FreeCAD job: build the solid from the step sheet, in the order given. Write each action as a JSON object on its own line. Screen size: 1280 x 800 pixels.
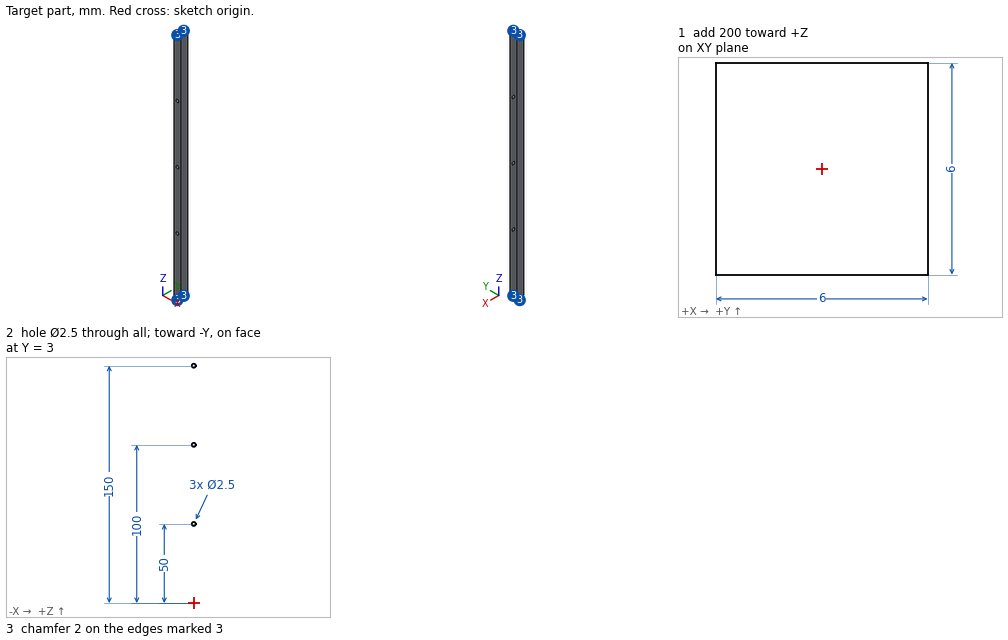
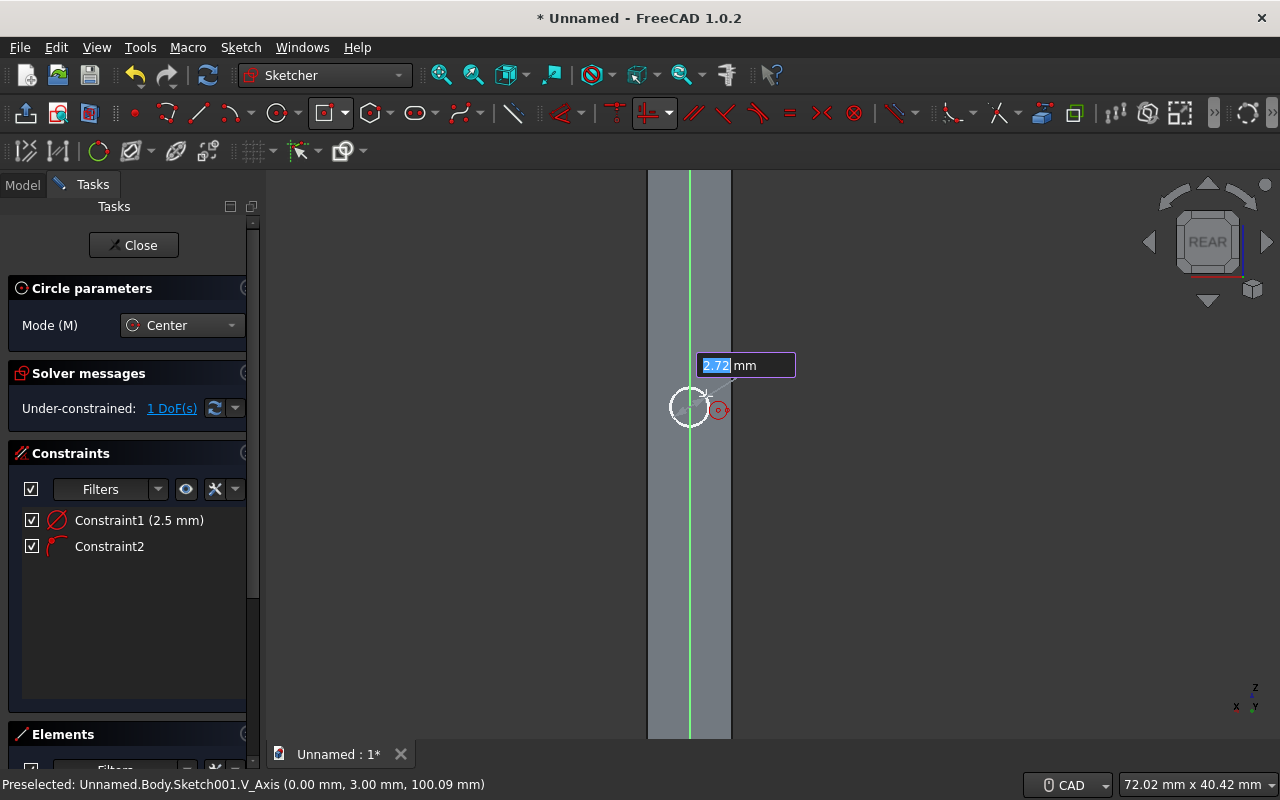
{"action": "type", "text": "2.5"}
{"action": "key", "text": "Return"}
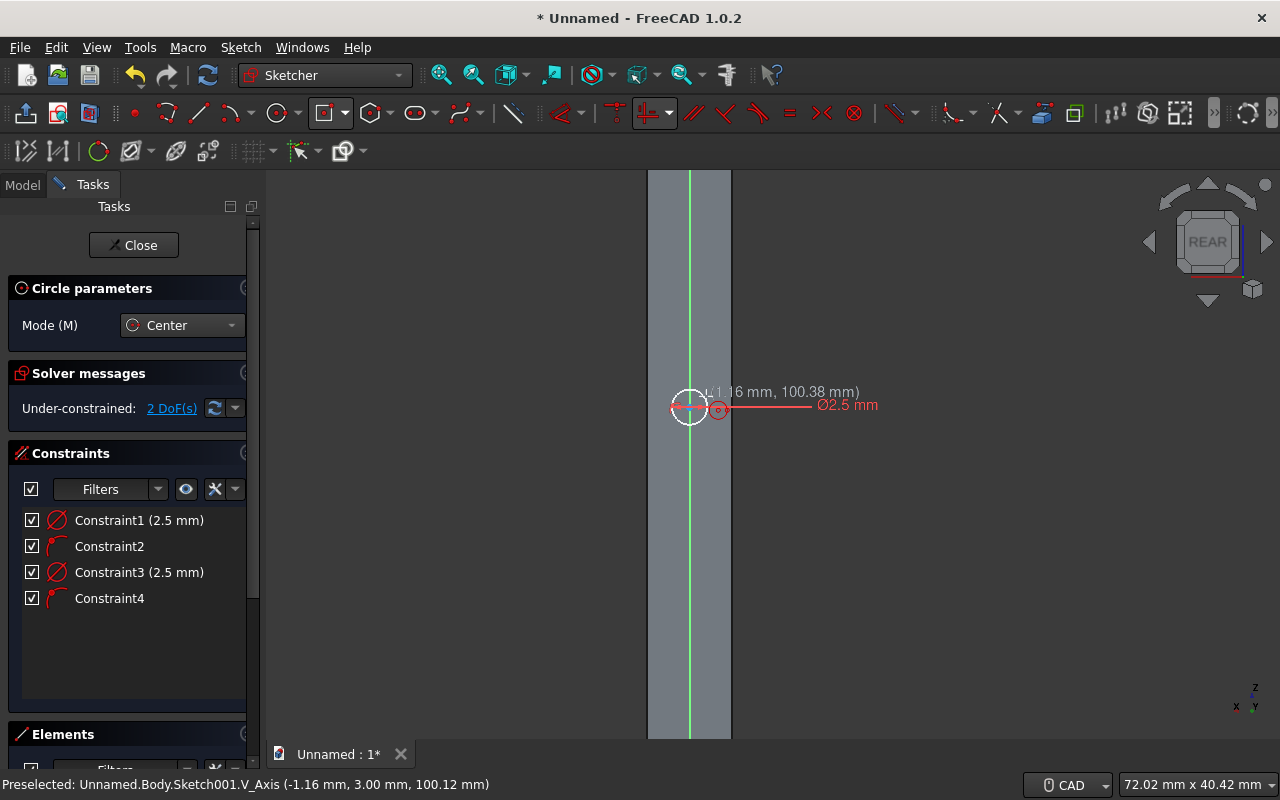
{"action": "scroll", "coordinate": [707, 397], "scroll_direction": "down", "scroll_amount": 9}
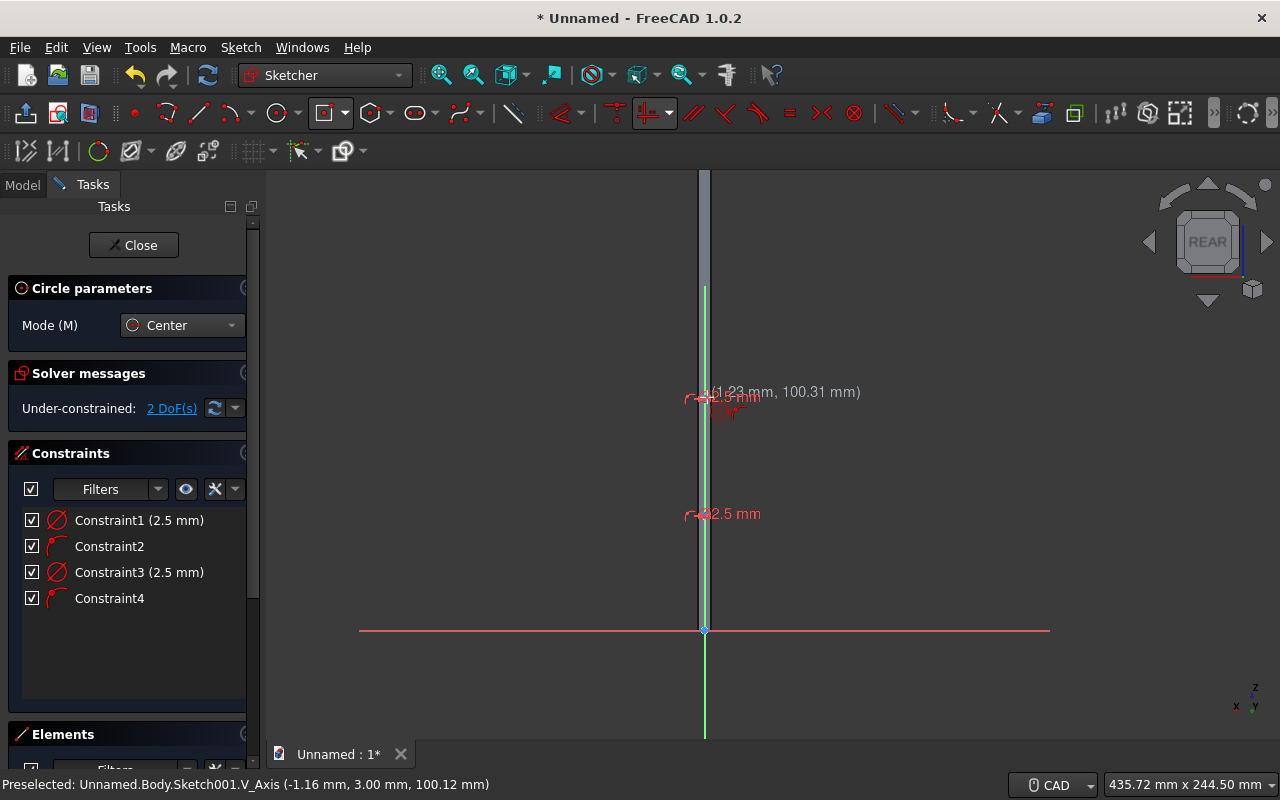
{"action": "scroll", "coordinate": [705, 282], "scroll_direction": "up", "scroll_amount": 11}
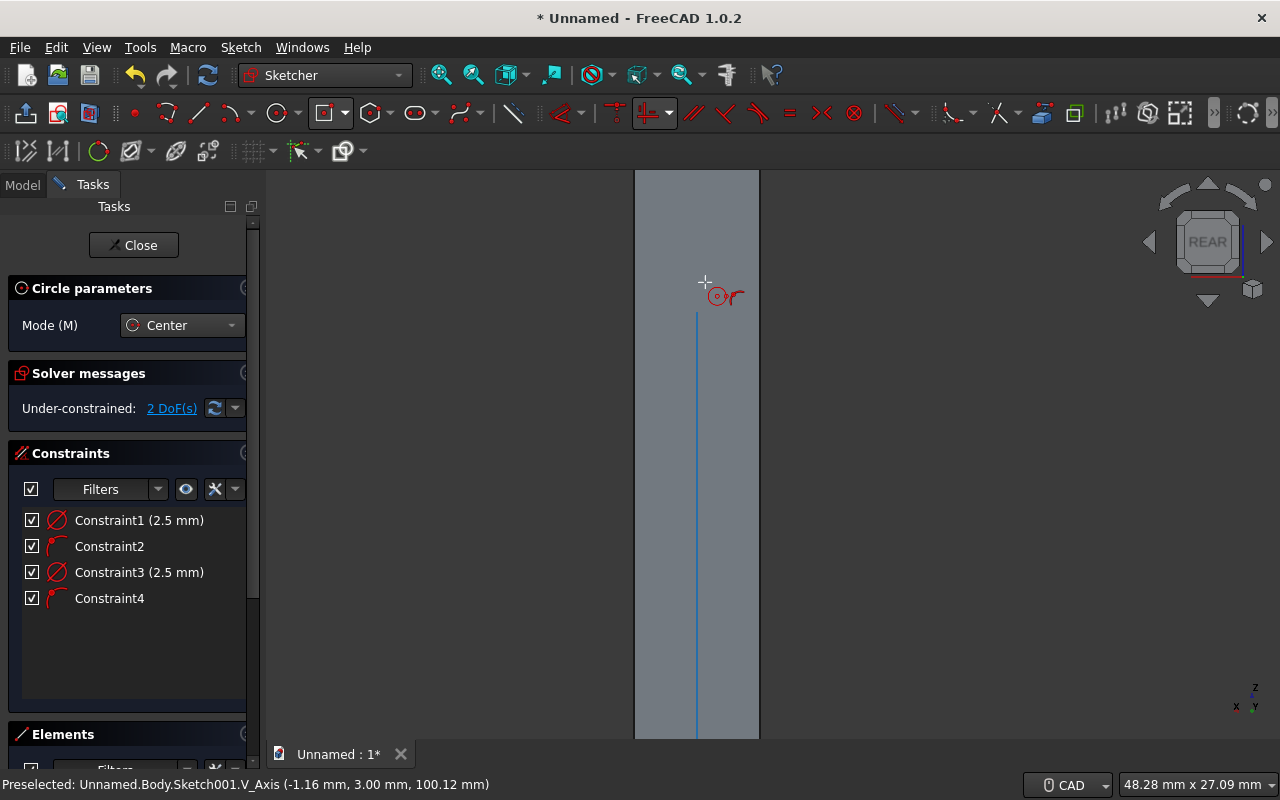
{"action": "scroll", "coordinate": [705, 282], "scroll_direction": "down", "scroll_amount": 11}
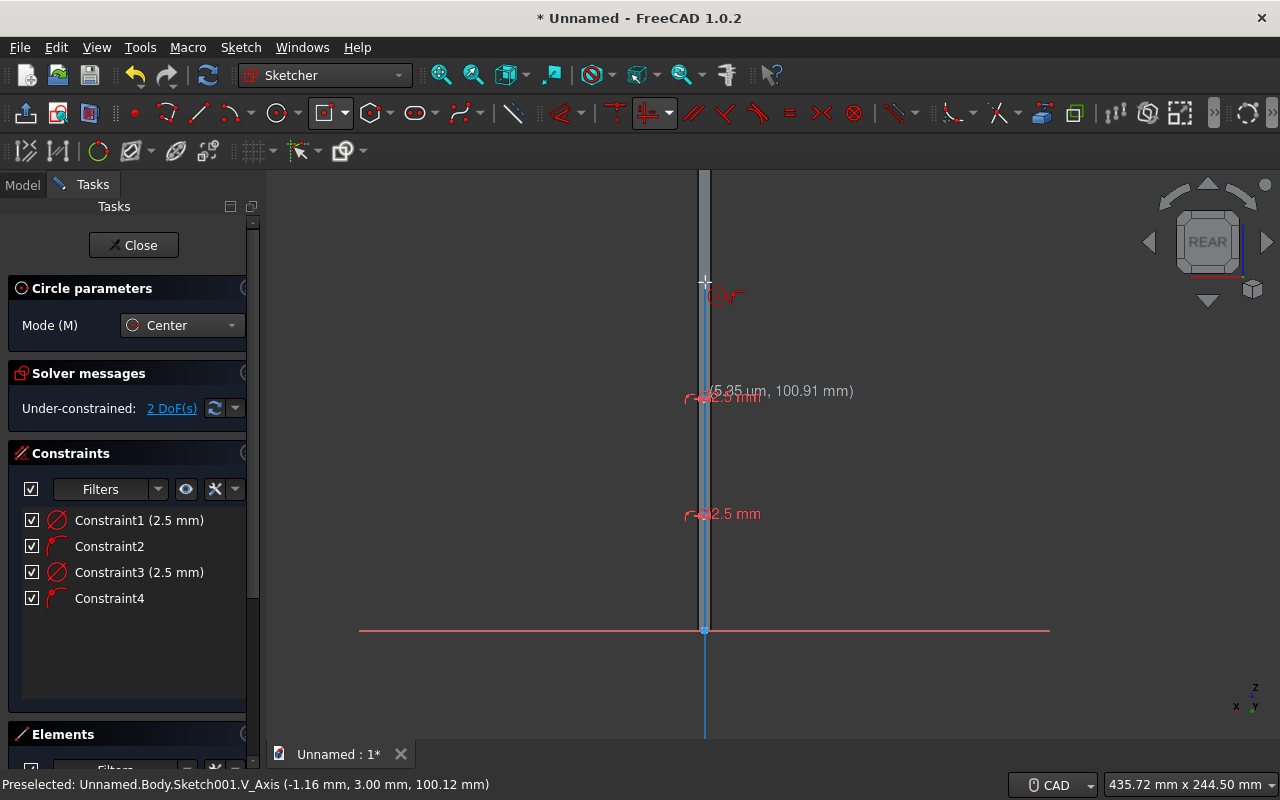
{"action": "left_click", "coordinate": [705, 282]}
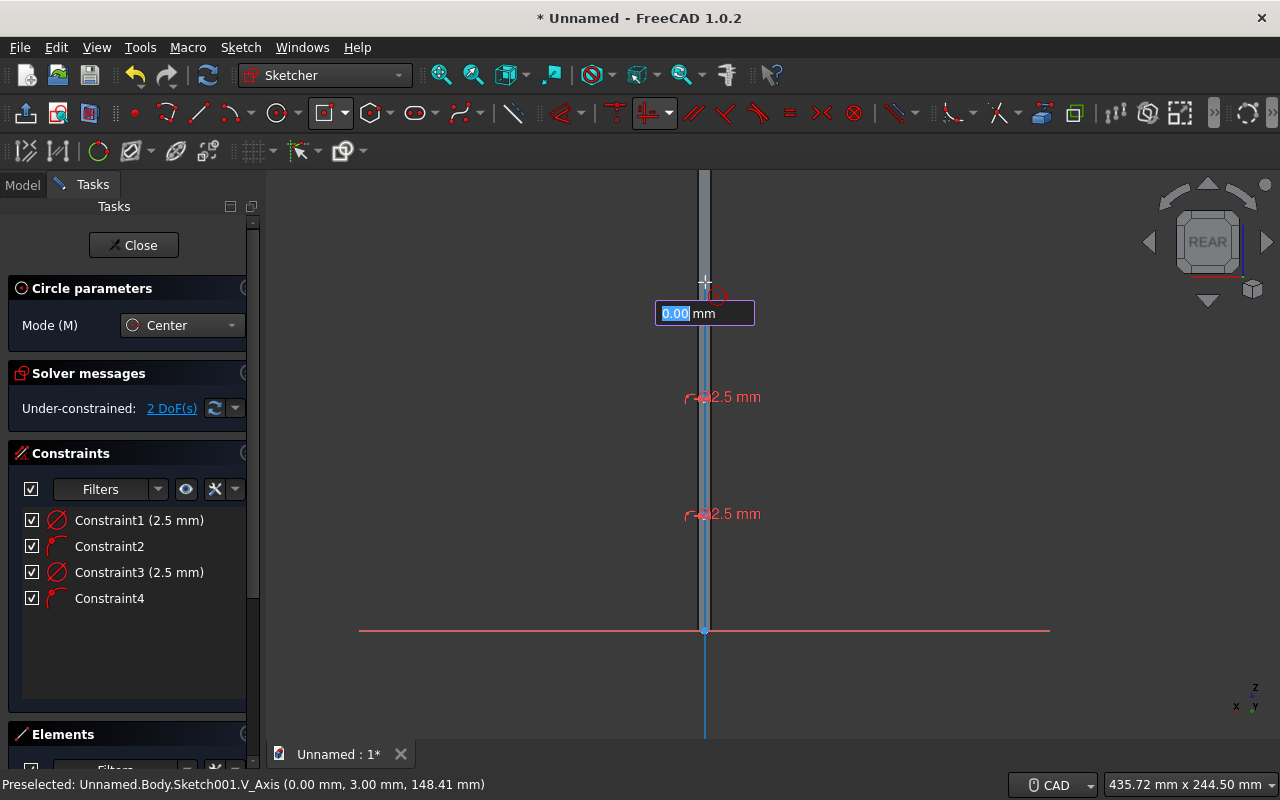
{"action": "scroll", "coordinate": [707, 281], "scroll_direction": "up", "scroll_amount": 9}
{"action": "mouse_move", "coordinate": [706, 279]}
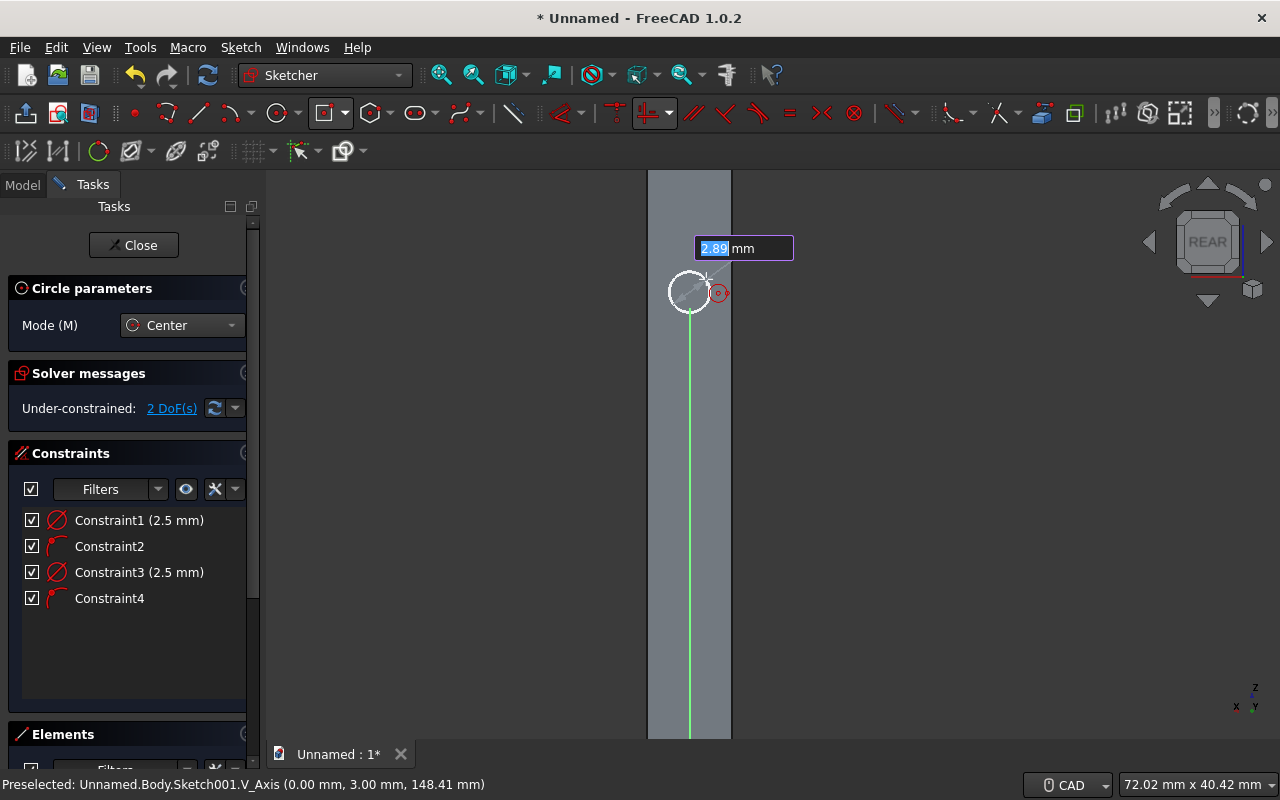
{"action": "type", "text": "2.5"}
{"action": "key", "text": "Return"}
{"action": "key", "text": "Escape"}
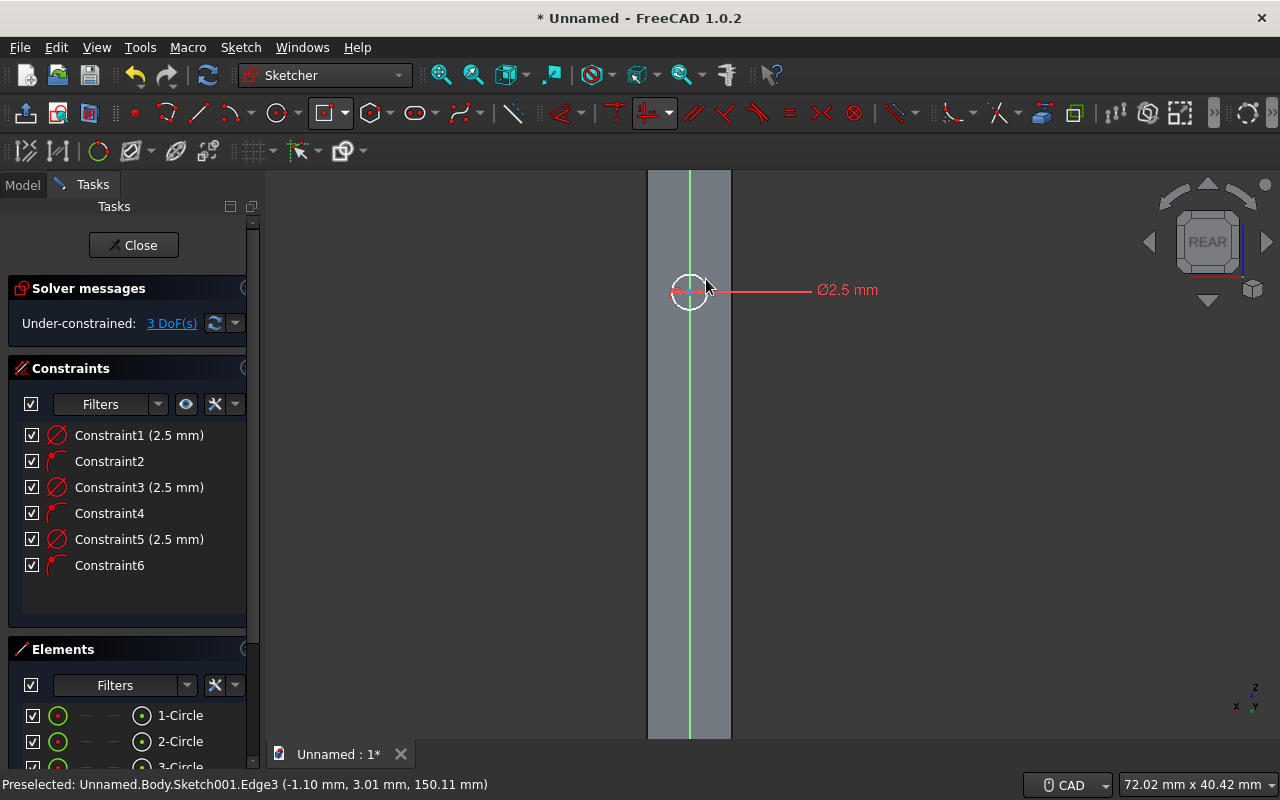
{"action": "left_click", "coordinate": [560, 114]}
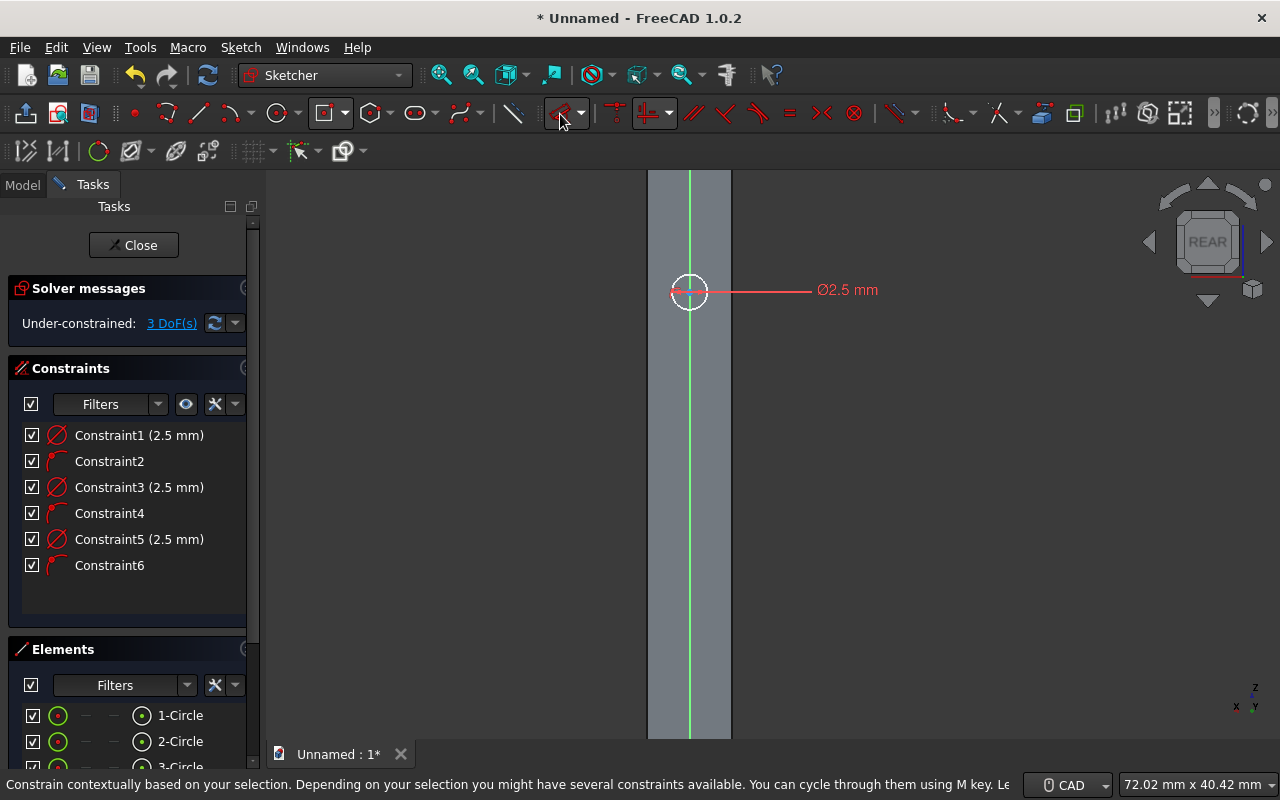
{"action": "scroll", "coordinate": [707, 281], "scroll_direction": "down", "scroll_amount": 9}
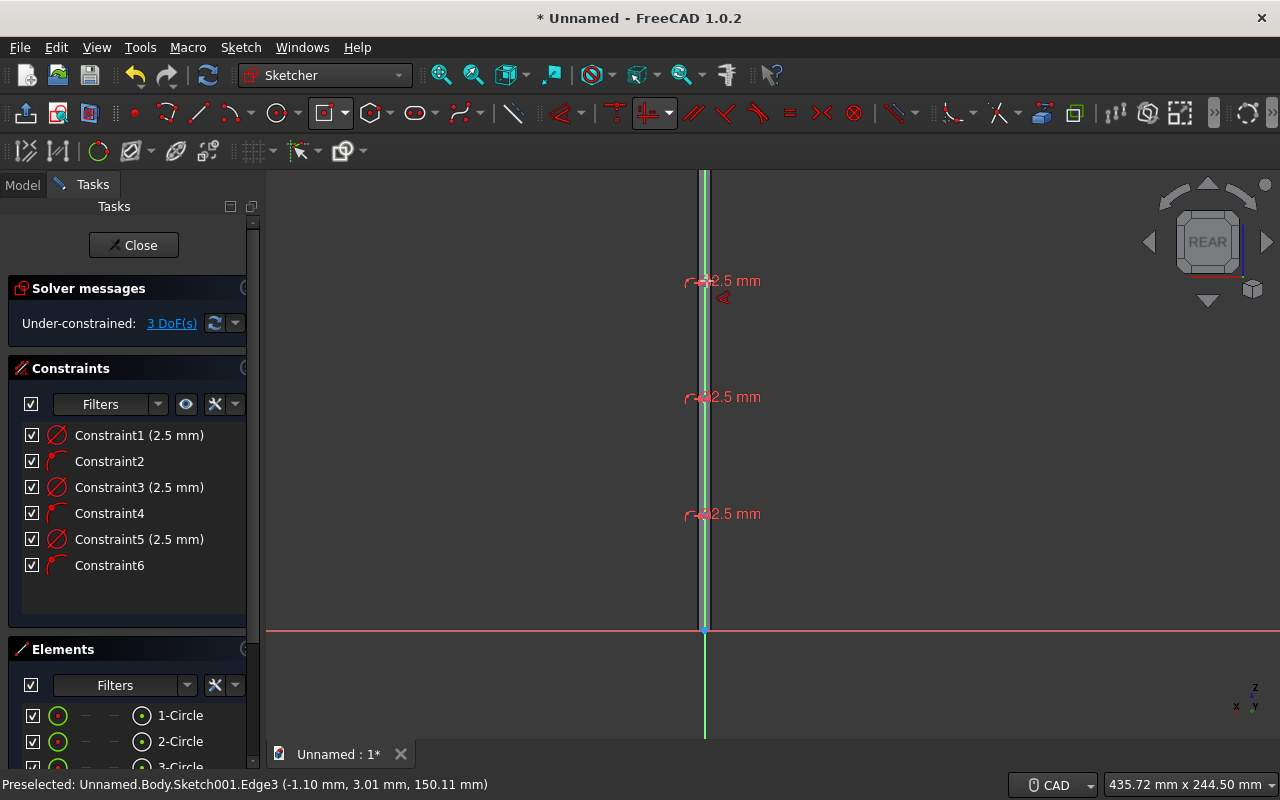
{"action": "left_click", "coordinate": [705, 516]}
{"action": "left_click", "coordinate": [739, 573]}